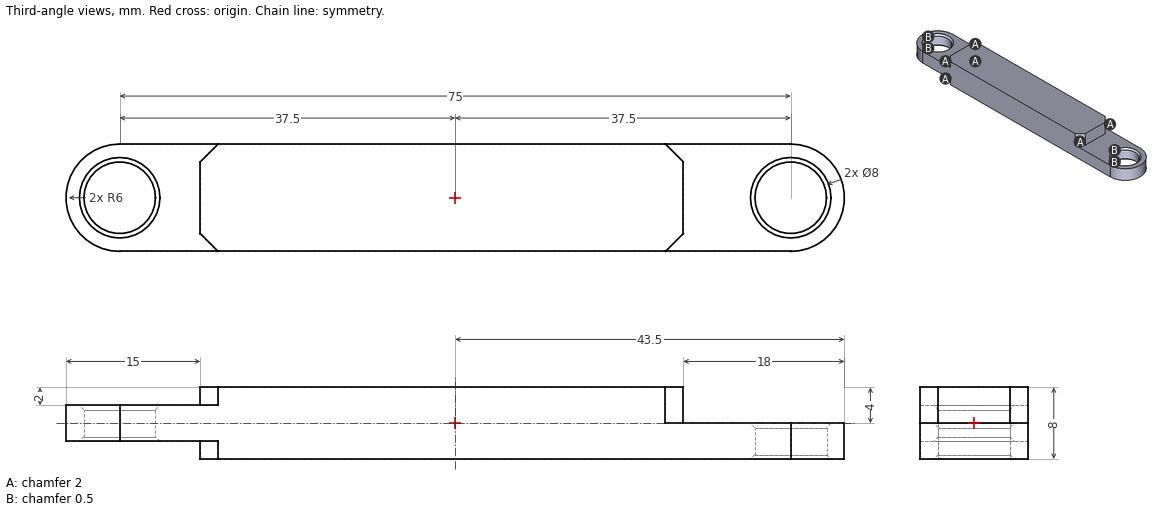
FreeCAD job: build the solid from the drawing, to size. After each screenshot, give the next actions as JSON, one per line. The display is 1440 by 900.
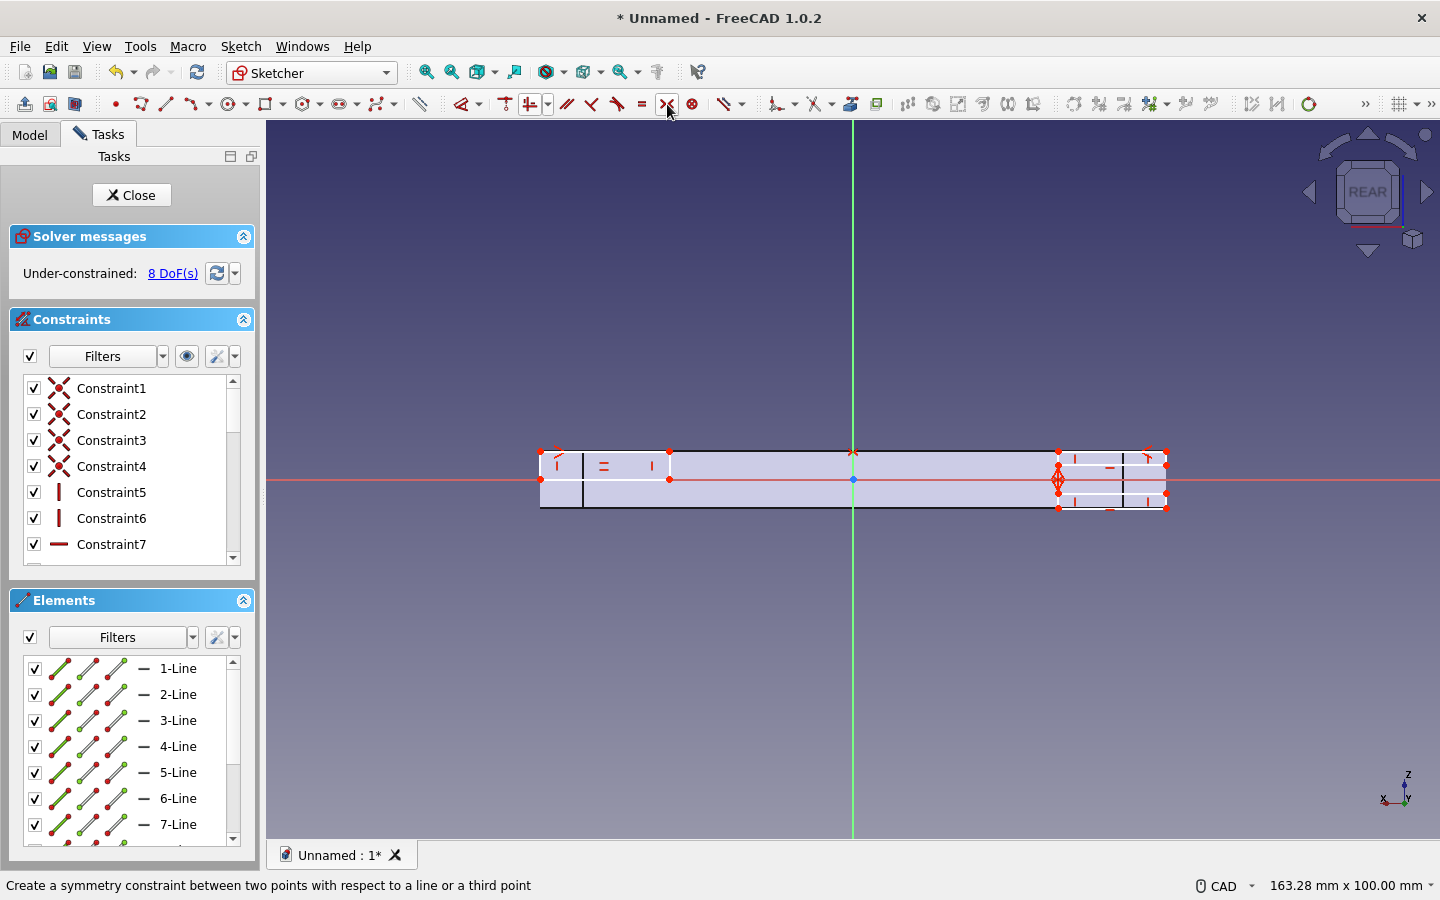
{"action": "left_click", "coordinate": [1166, 452]}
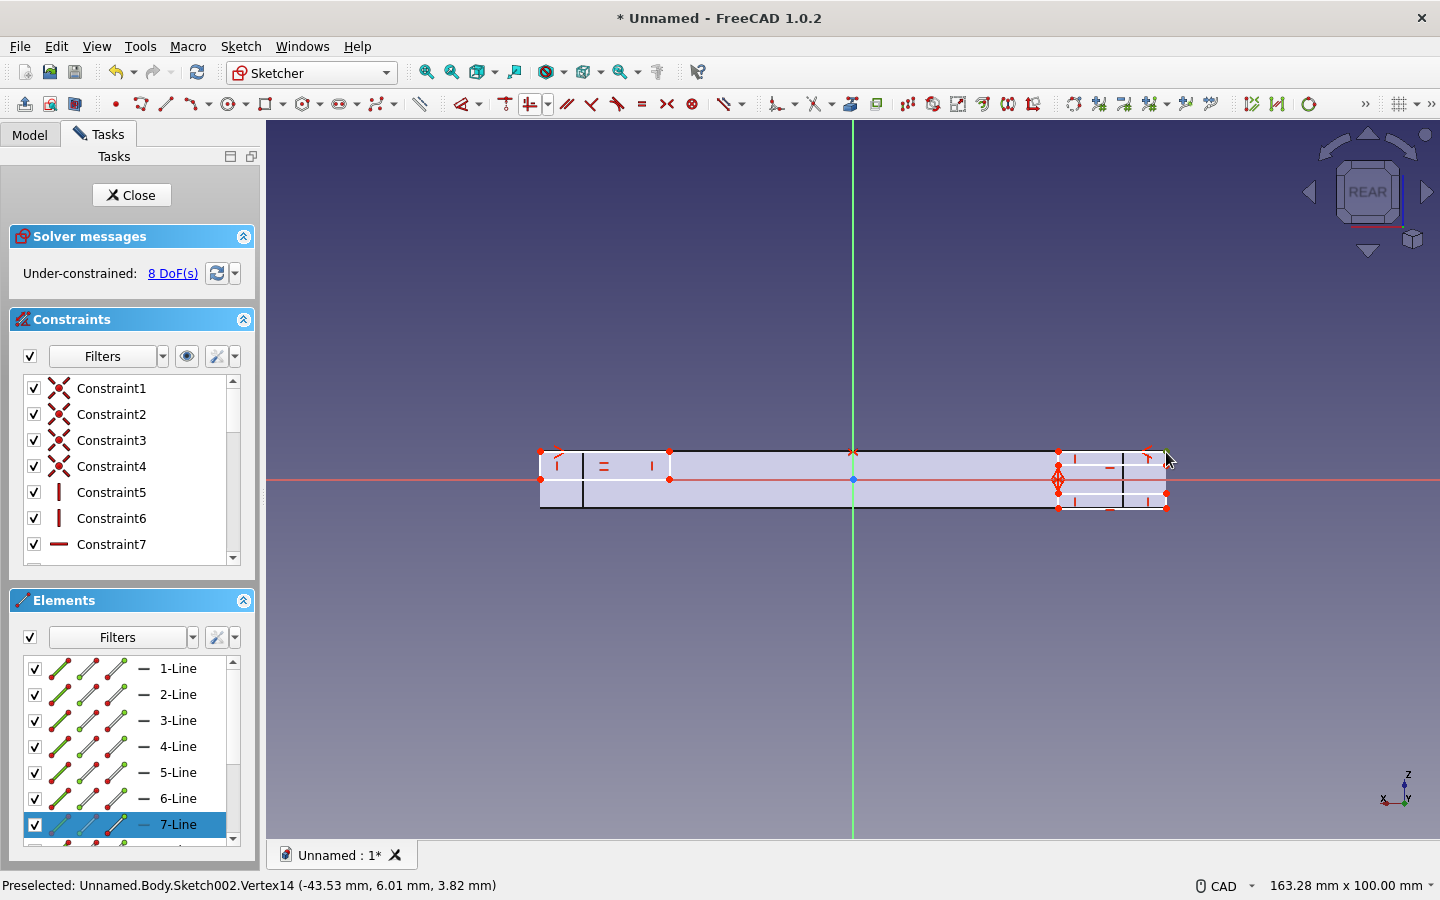
{"action": "left_click", "coordinate": [1166, 509]}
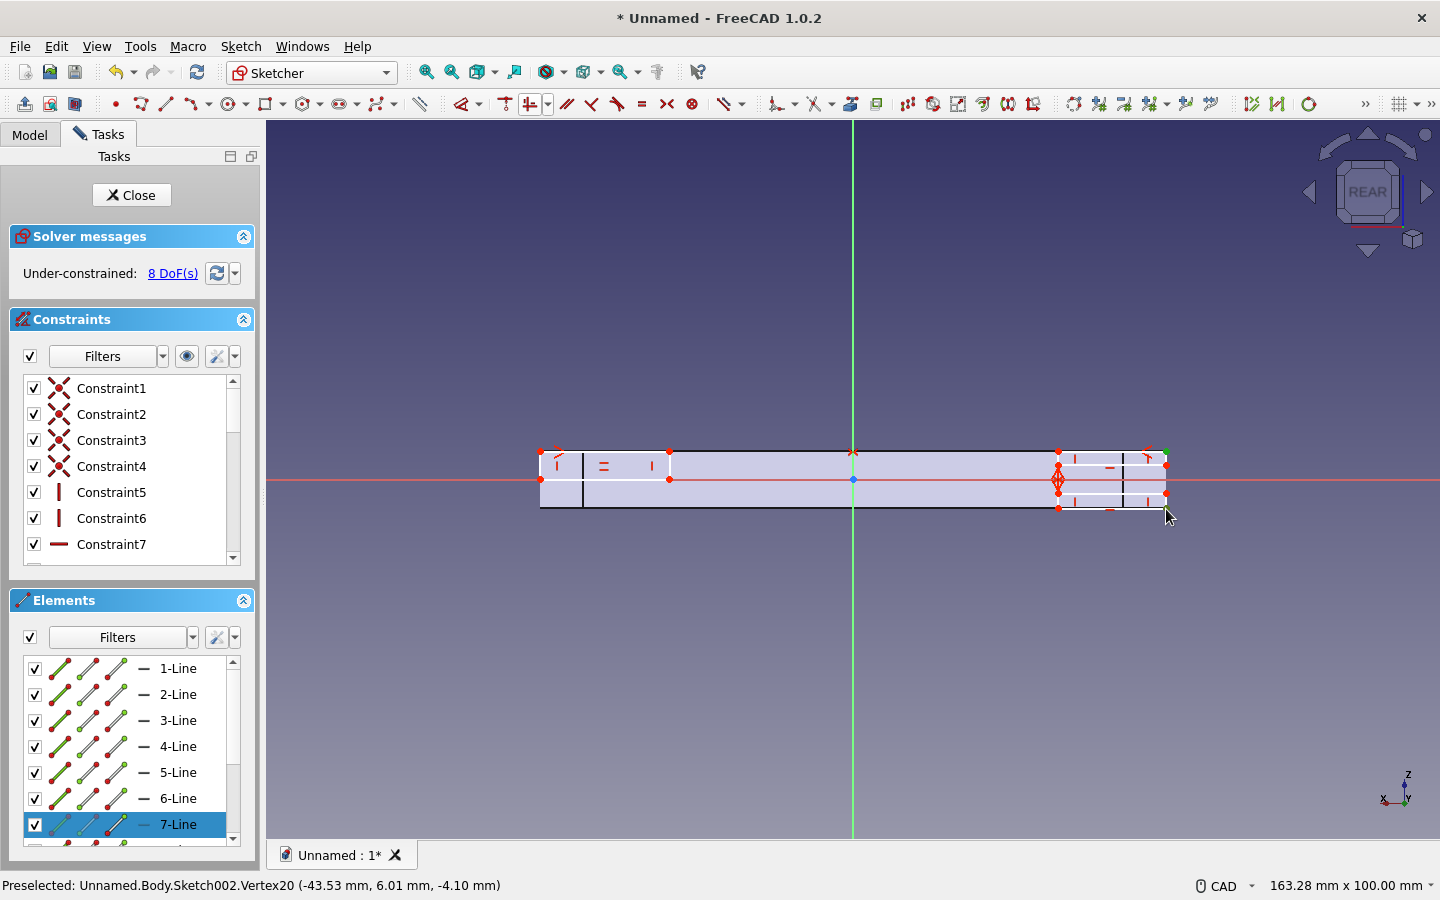
{"action": "left_click", "coordinate": [364, 479]}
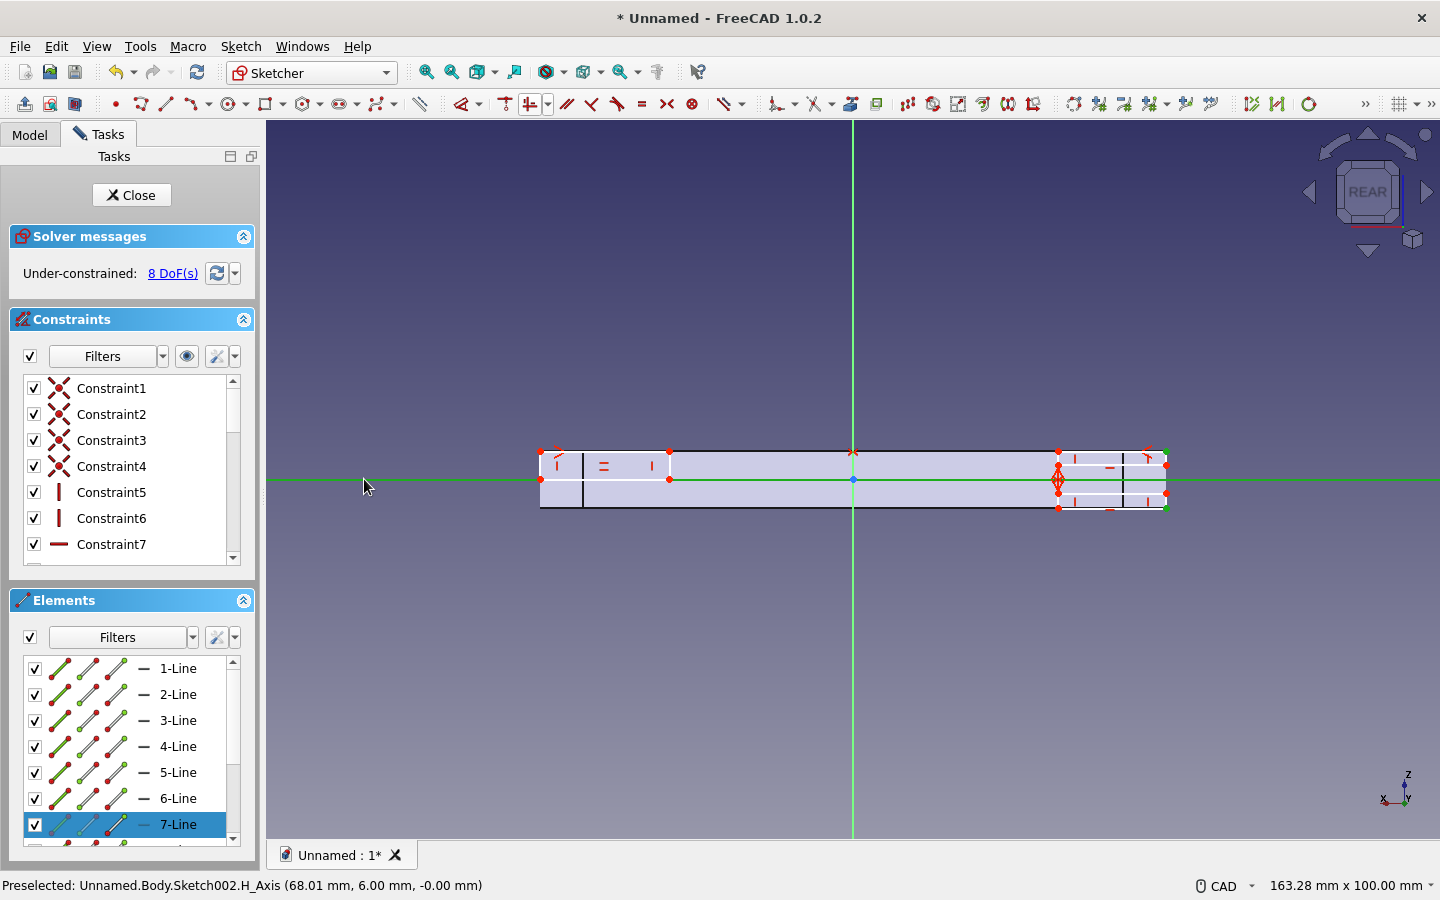
{"action": "left_click", "coordinate": [667, 104]}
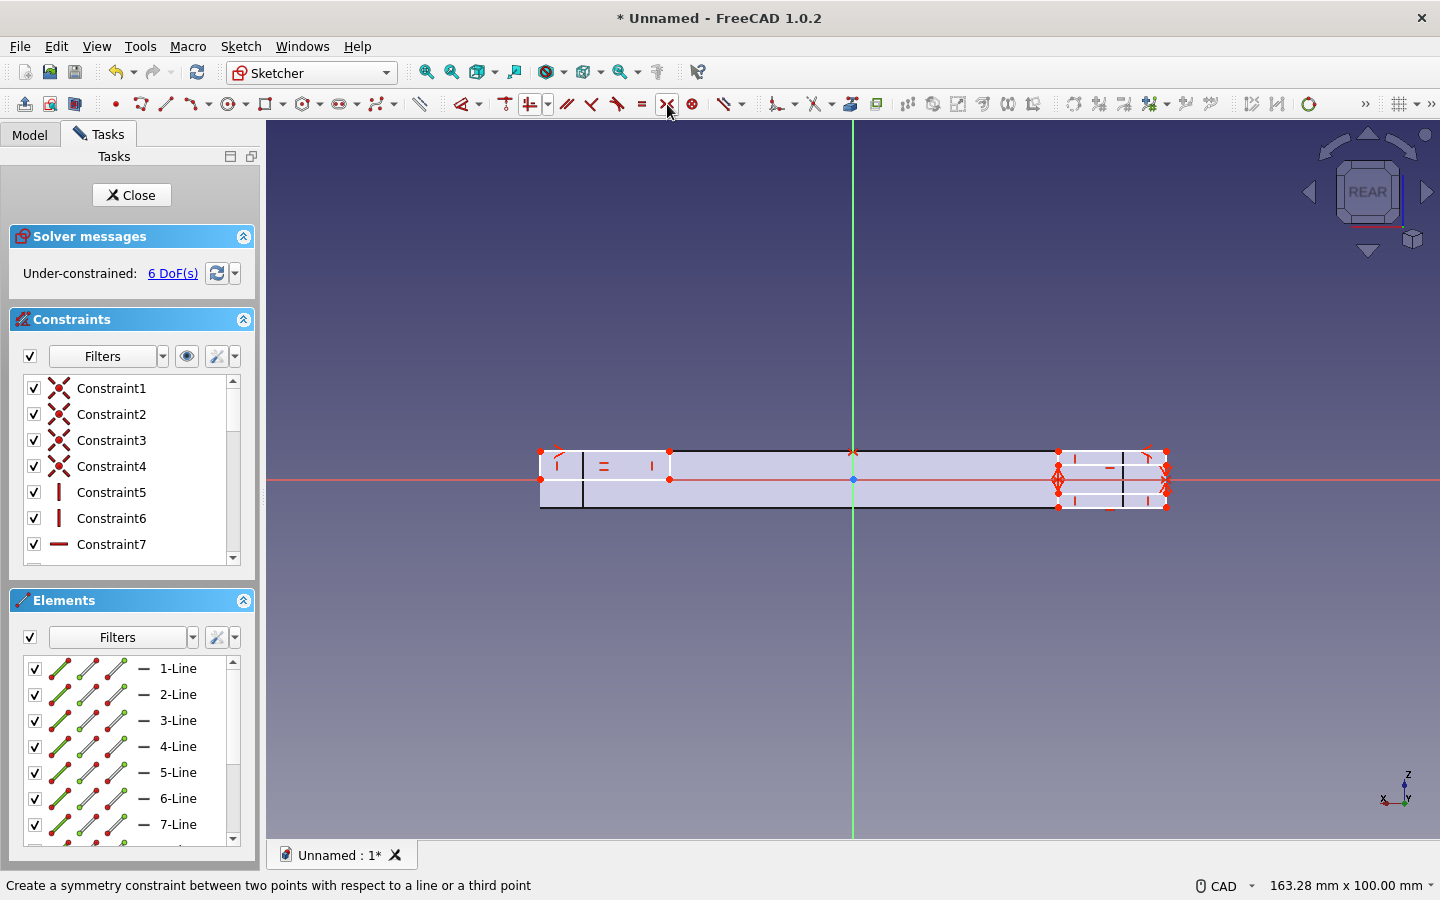
{"action": "left_click", "coordinate": [540, 480]}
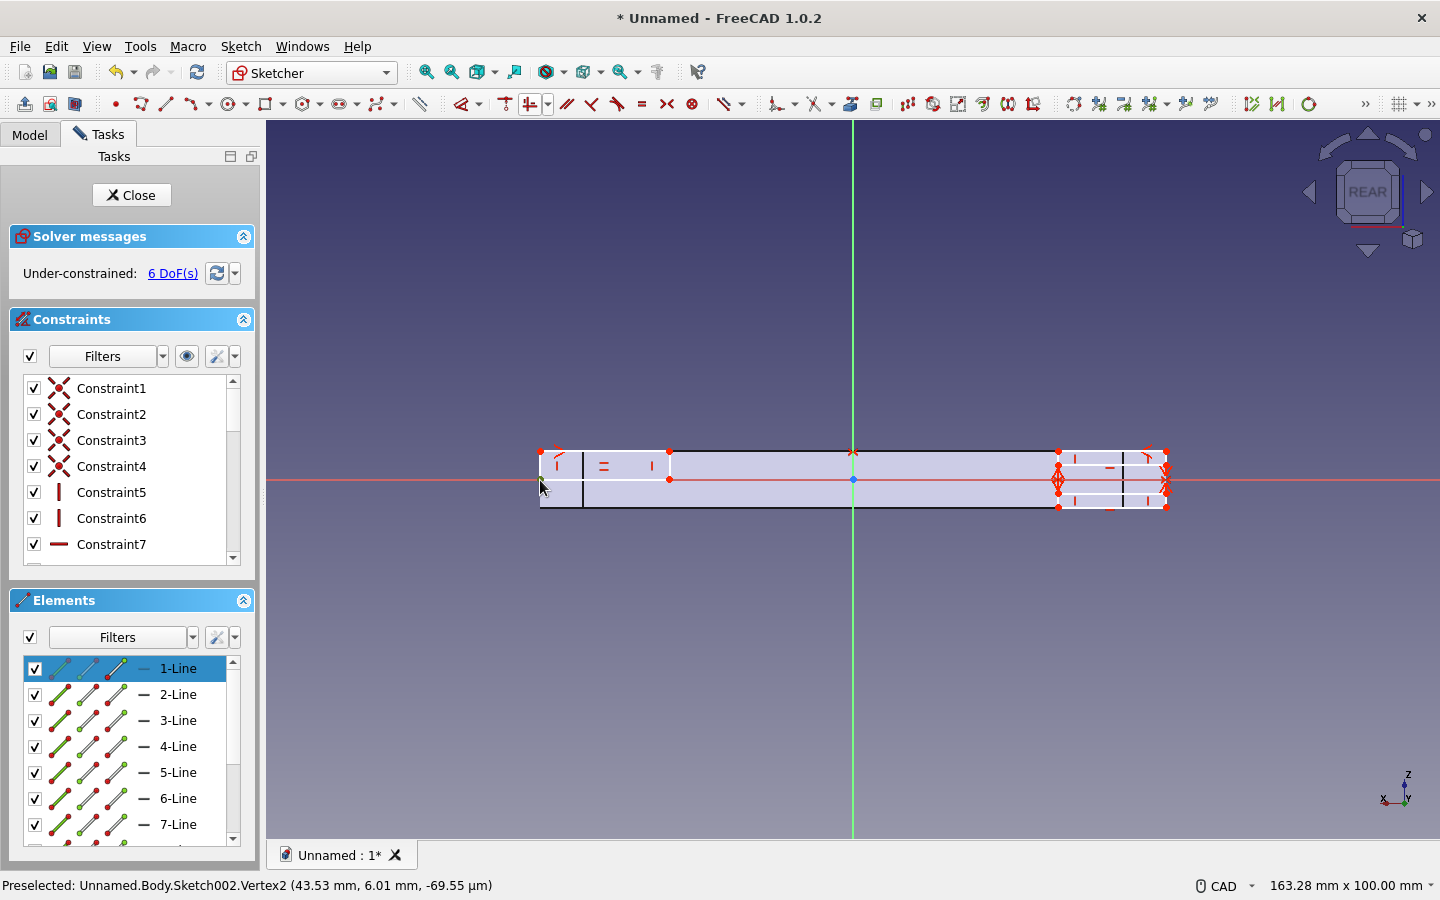
{"action": "left_click", "coordinate": [364, 479]}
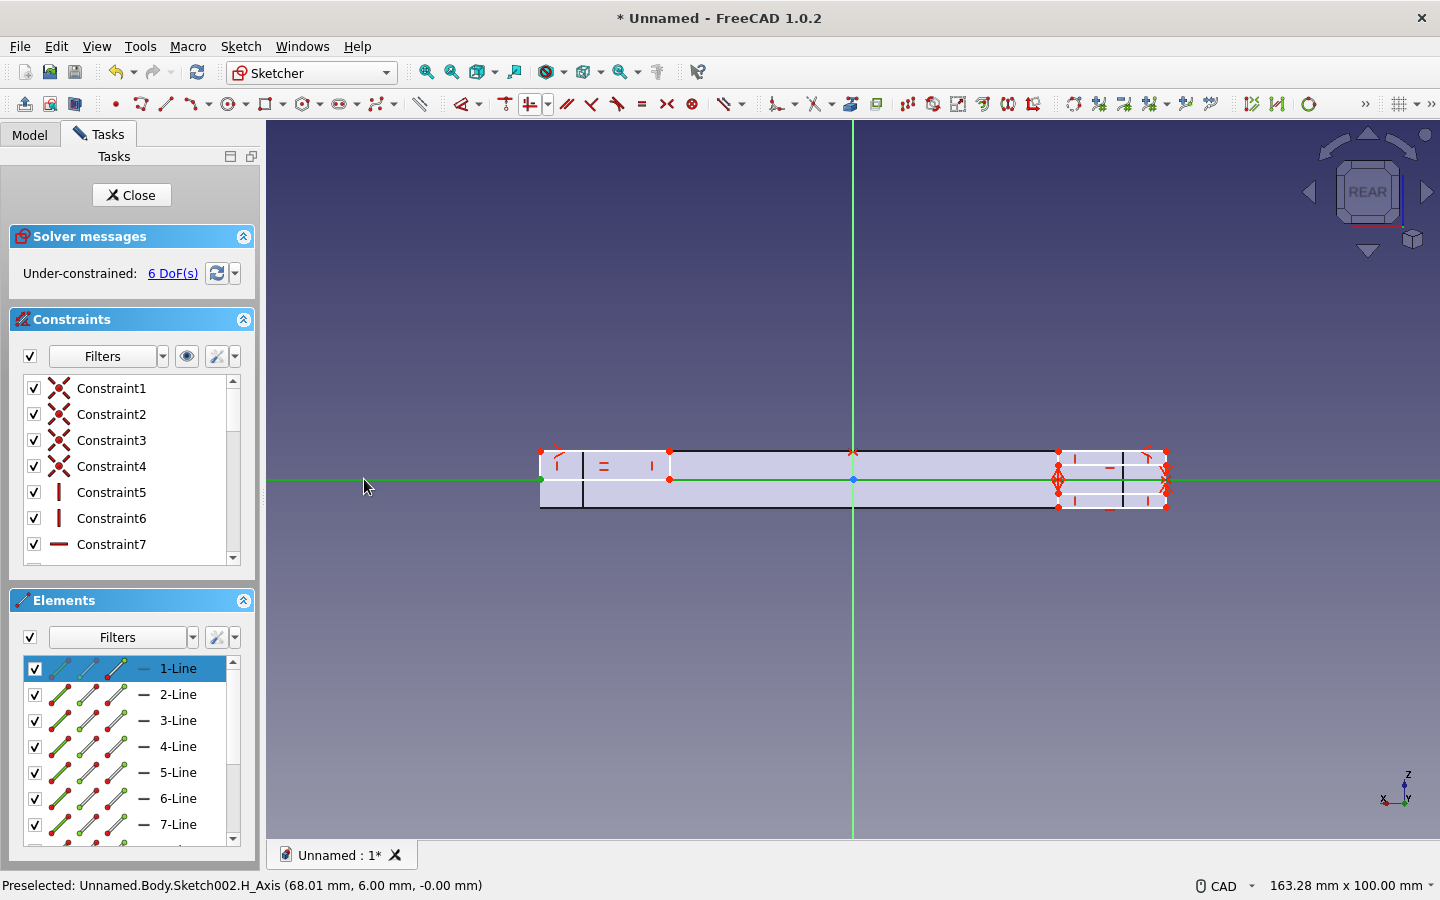
{"action": "left_click", "coordinate": [505, 104]}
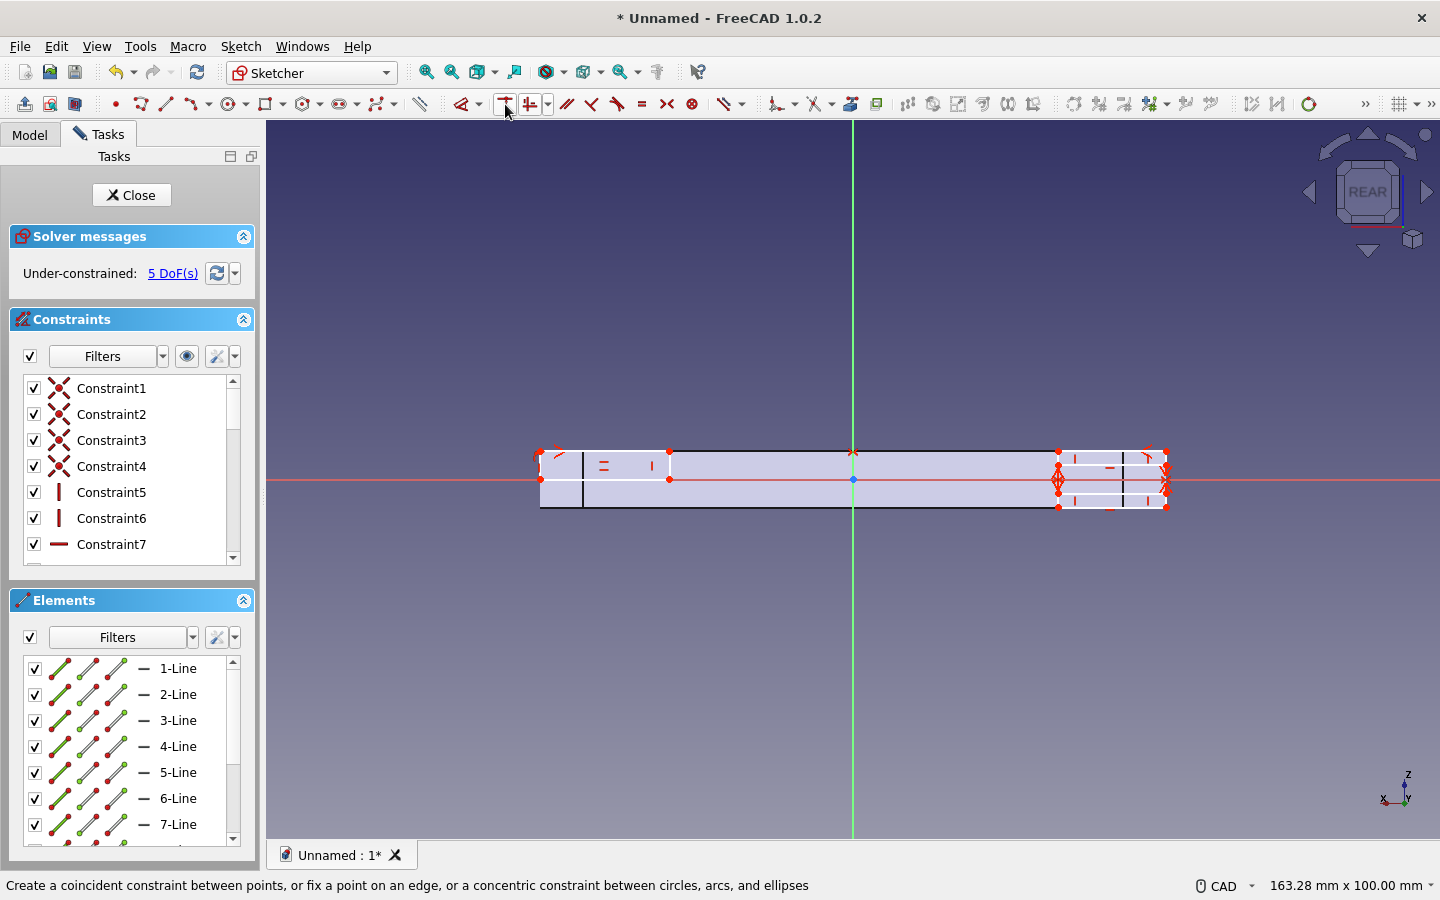
{"action": "left_click", "coordinate": [460, 104]}